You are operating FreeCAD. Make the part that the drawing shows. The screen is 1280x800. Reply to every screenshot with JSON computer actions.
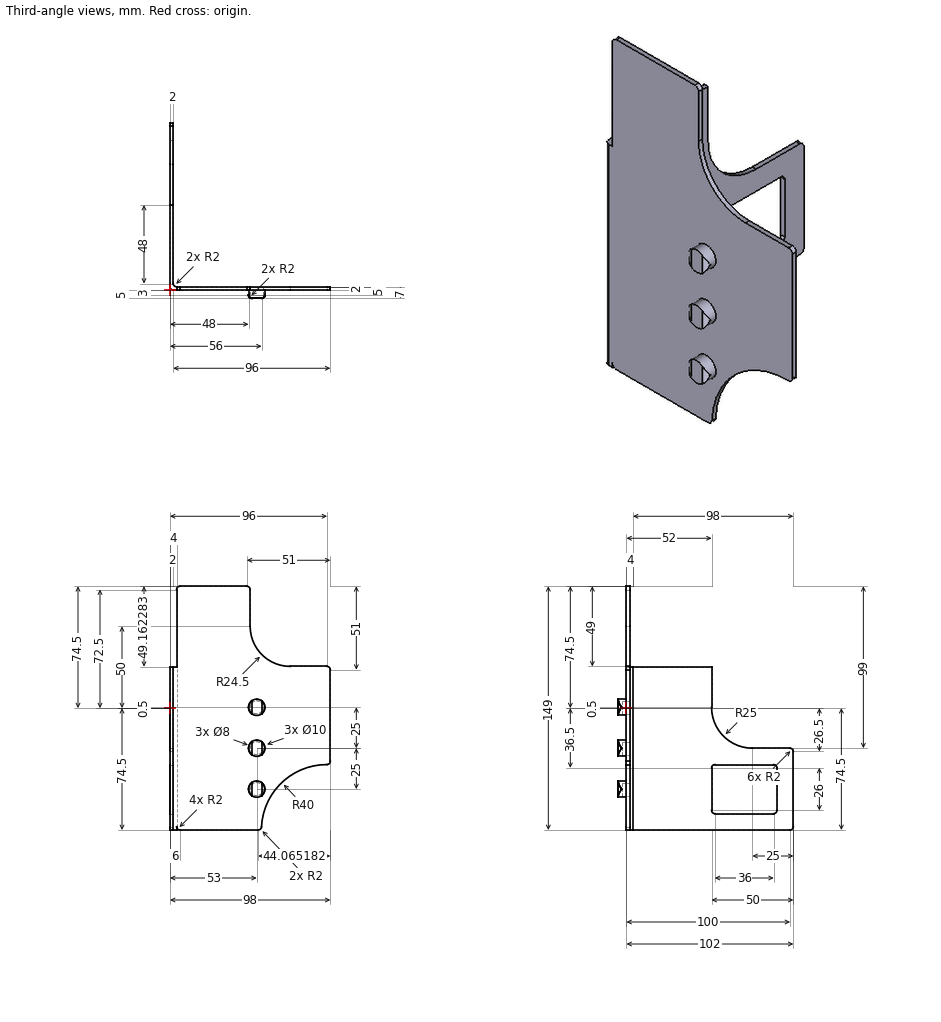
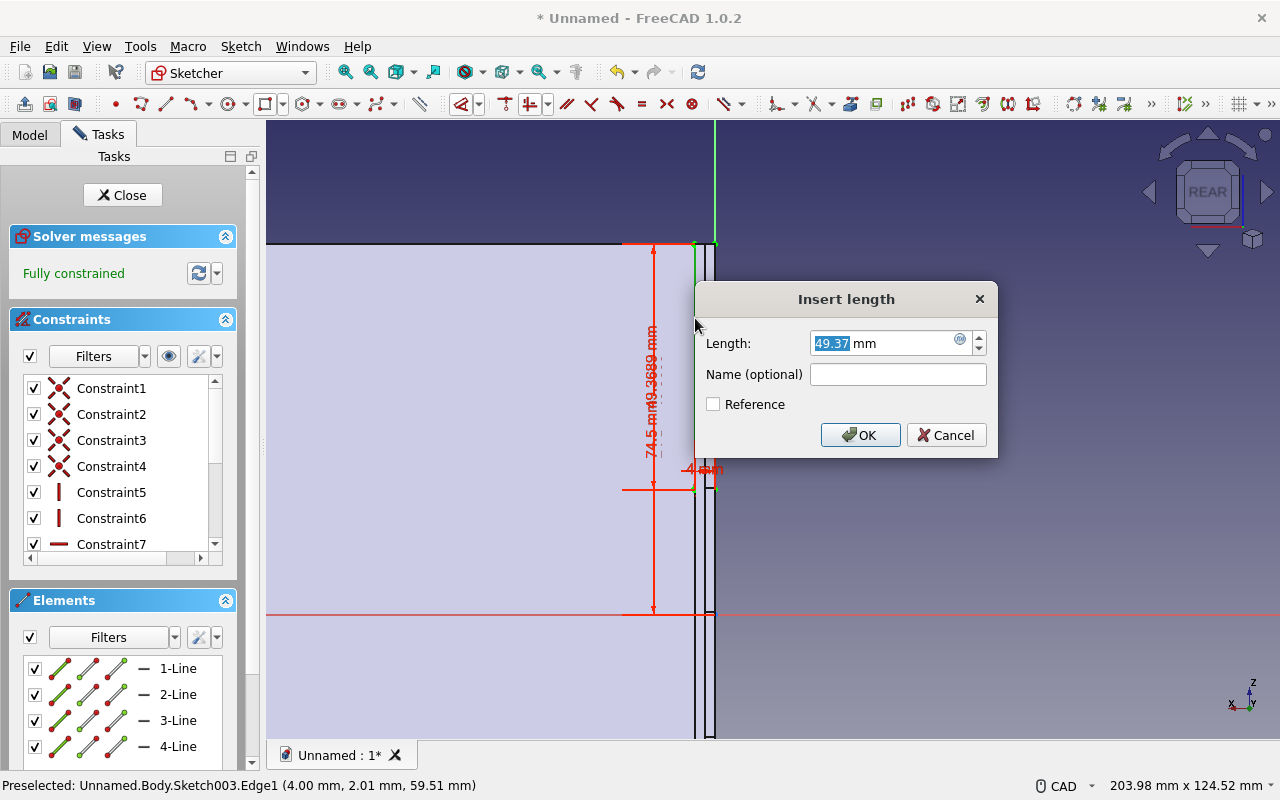
{"action": "type", "text": "49.162283"}
{"action": "key", "text": "Return"}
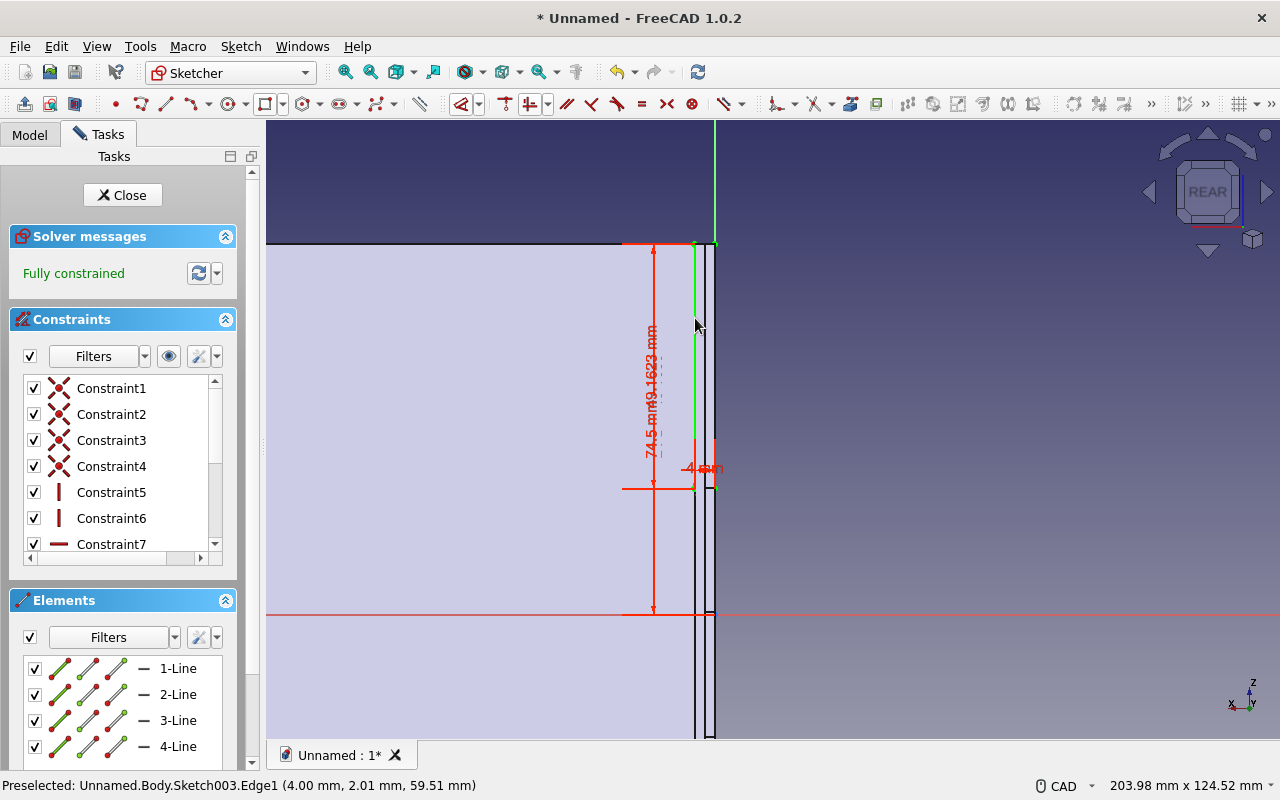
{"action": "left_click", "coordinate": [123, 195]}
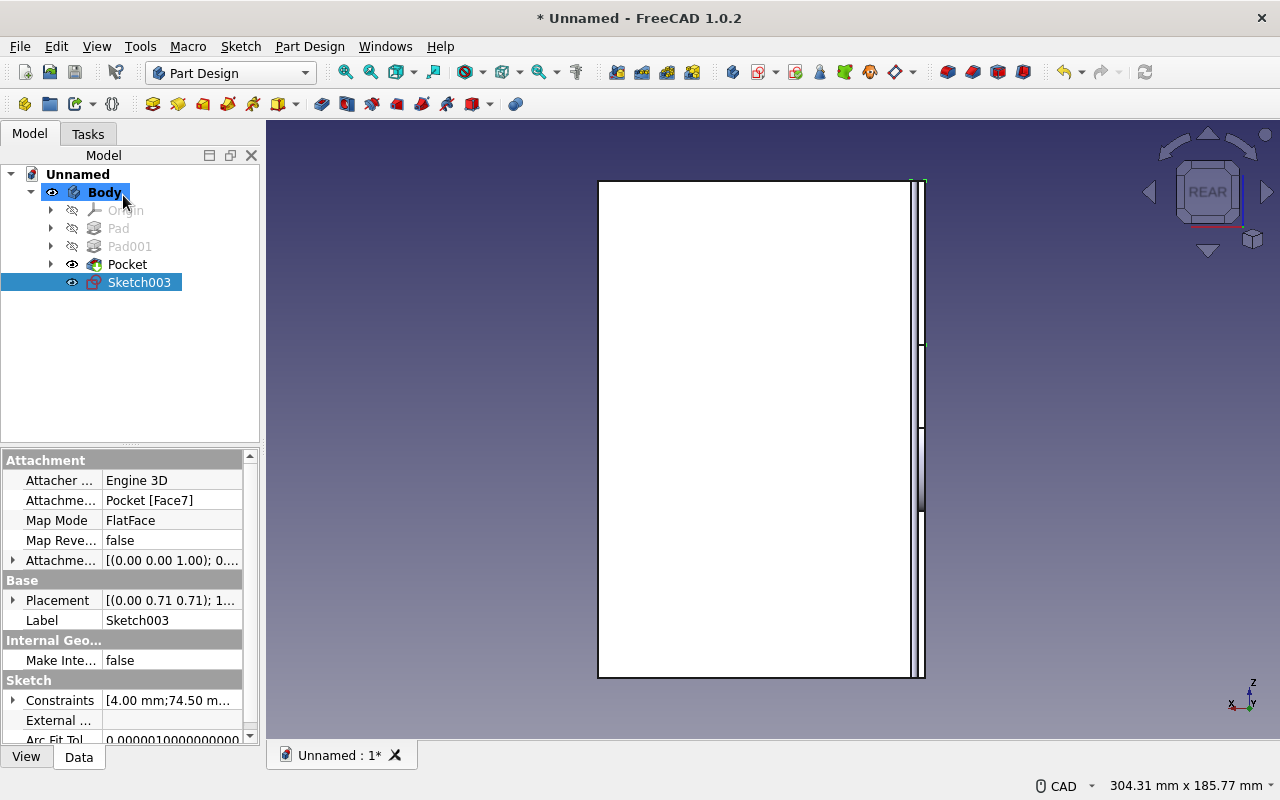
{"action": "left_click", "coordinate": [322, 104]}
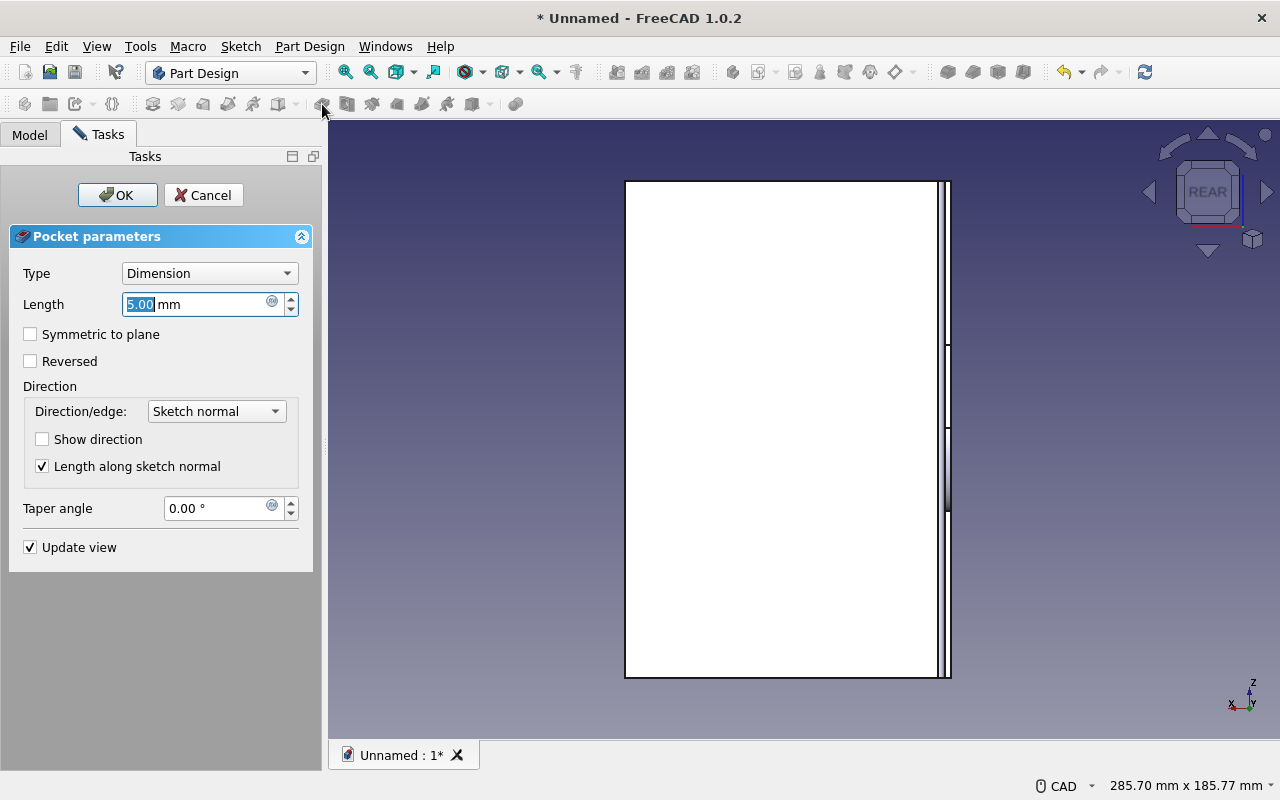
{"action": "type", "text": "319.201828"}
{"action": "key", "text": "Tab"}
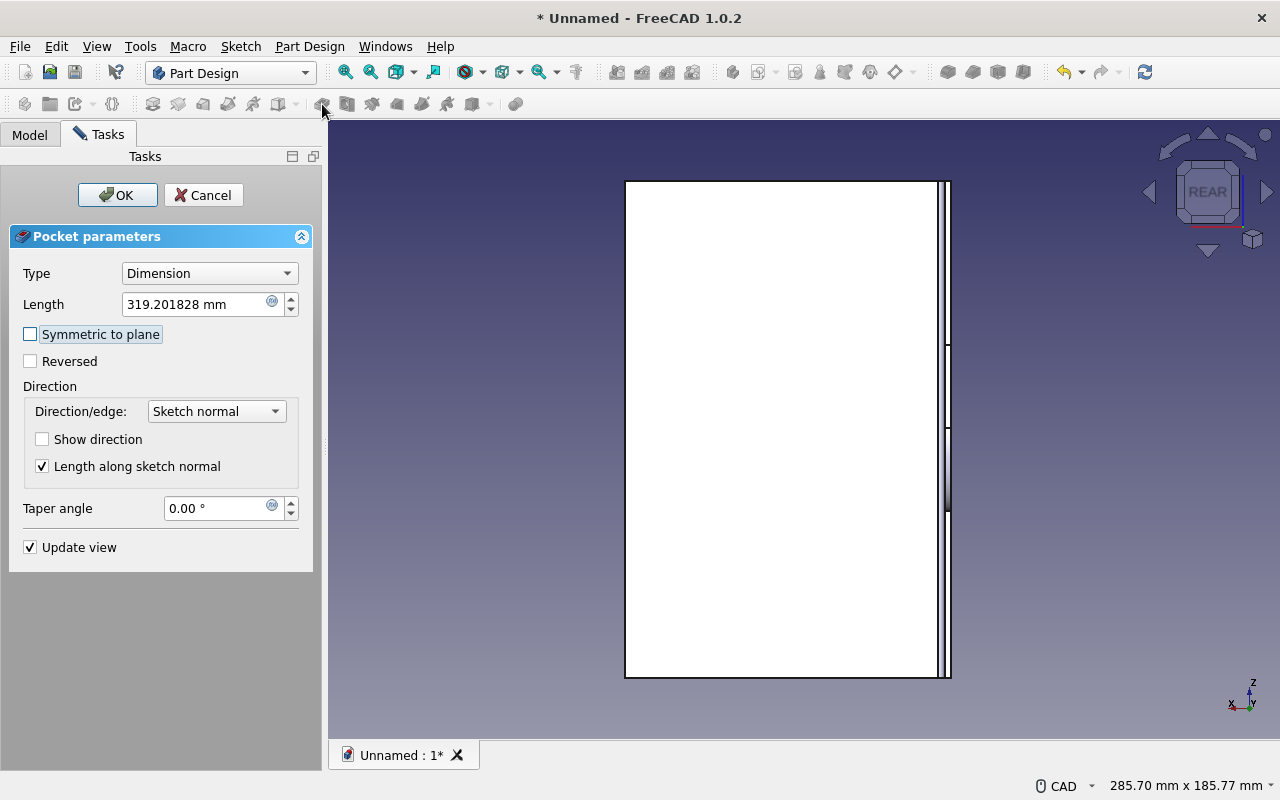
{"action": "left_click", "coordinate": [31, 334]}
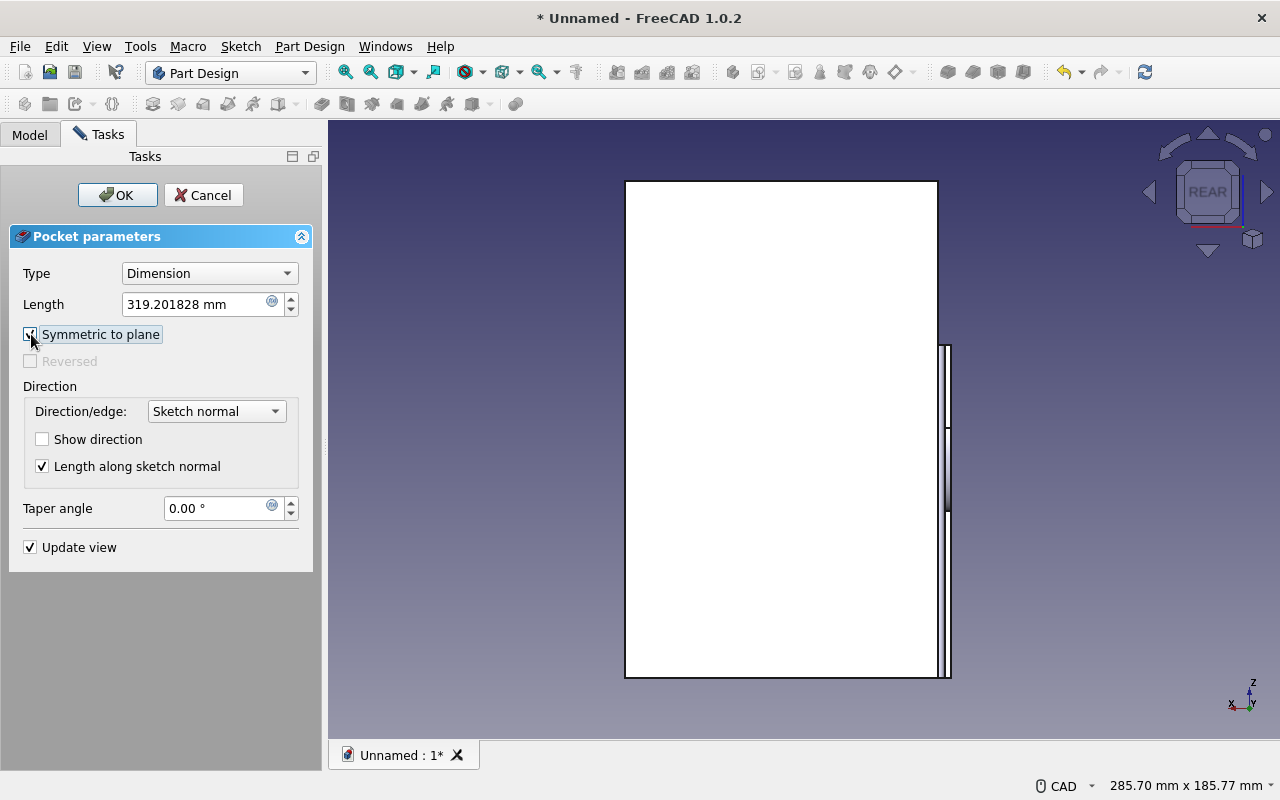
{"action": "left_click", "coordinate": [118, 195]}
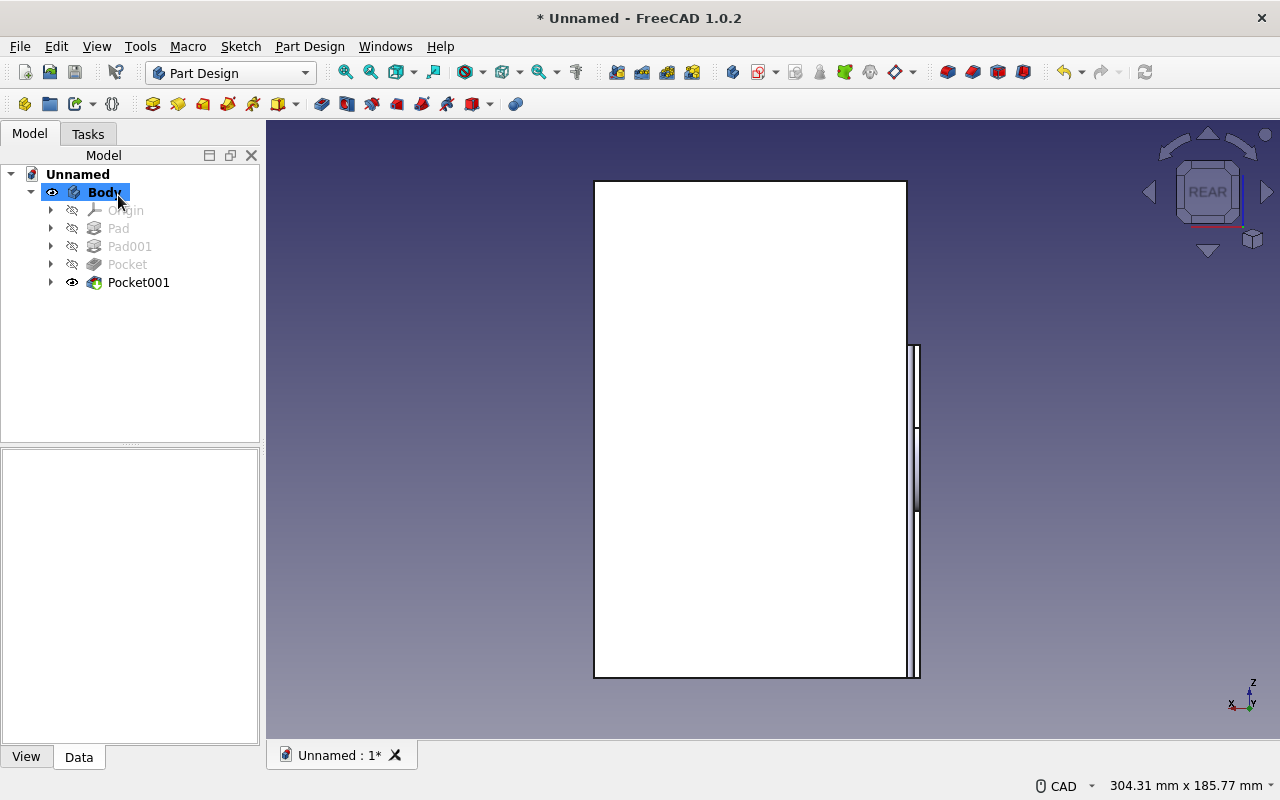
{"action": "key", "text": "0"}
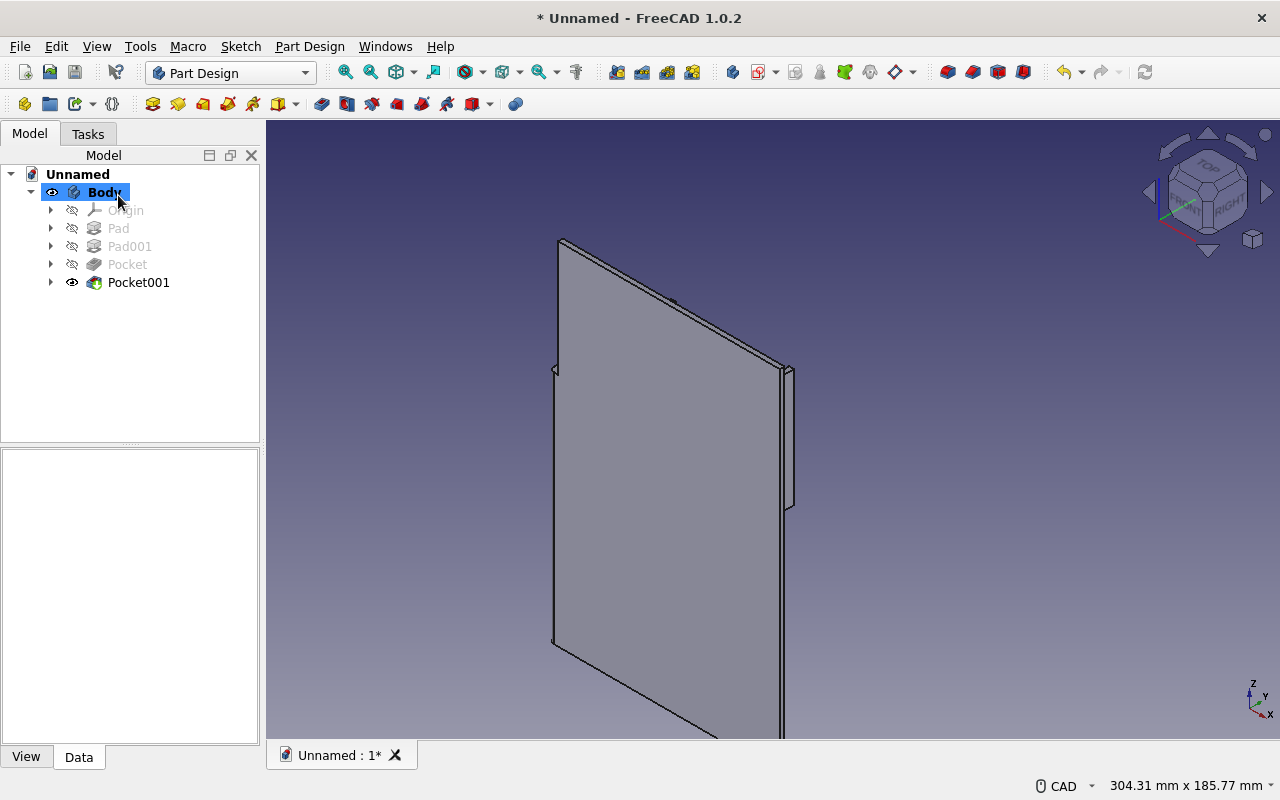
{"action": "key", "text": "v f"}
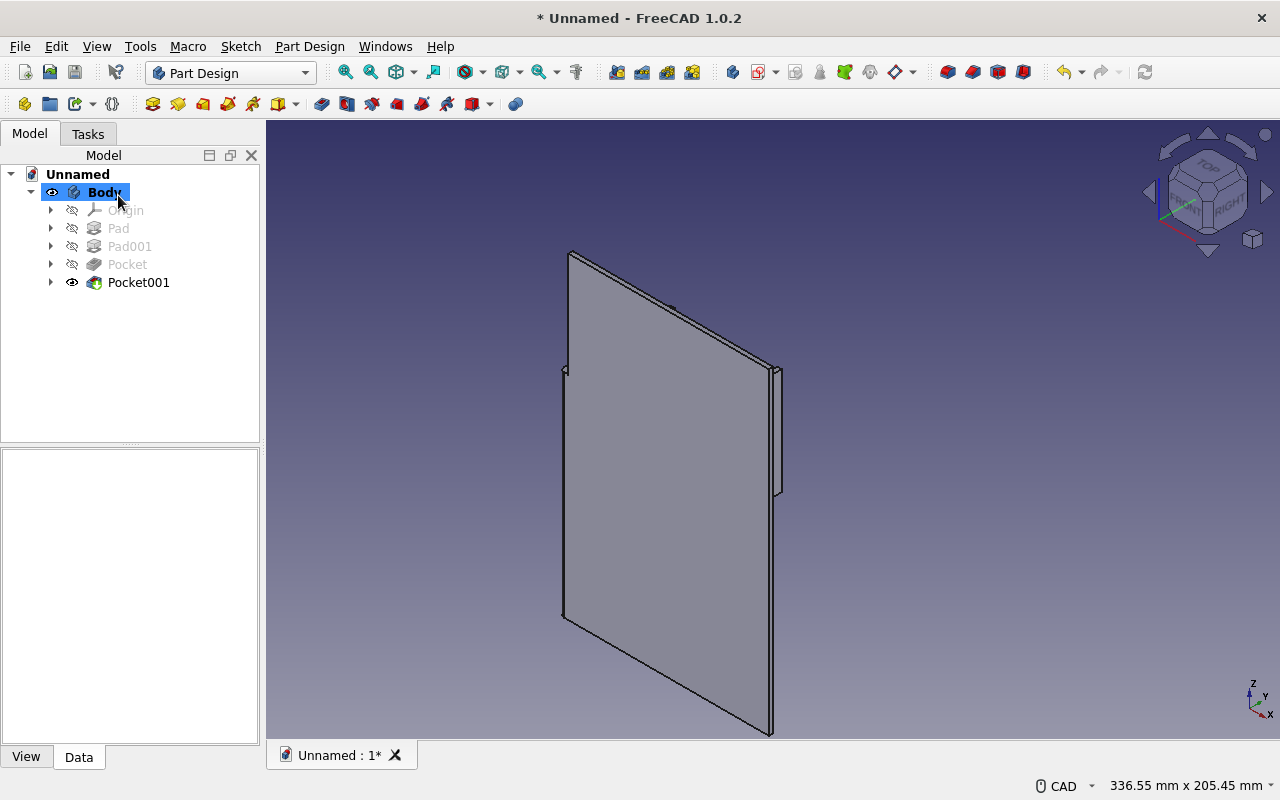
{"action": "key", "text": "3"}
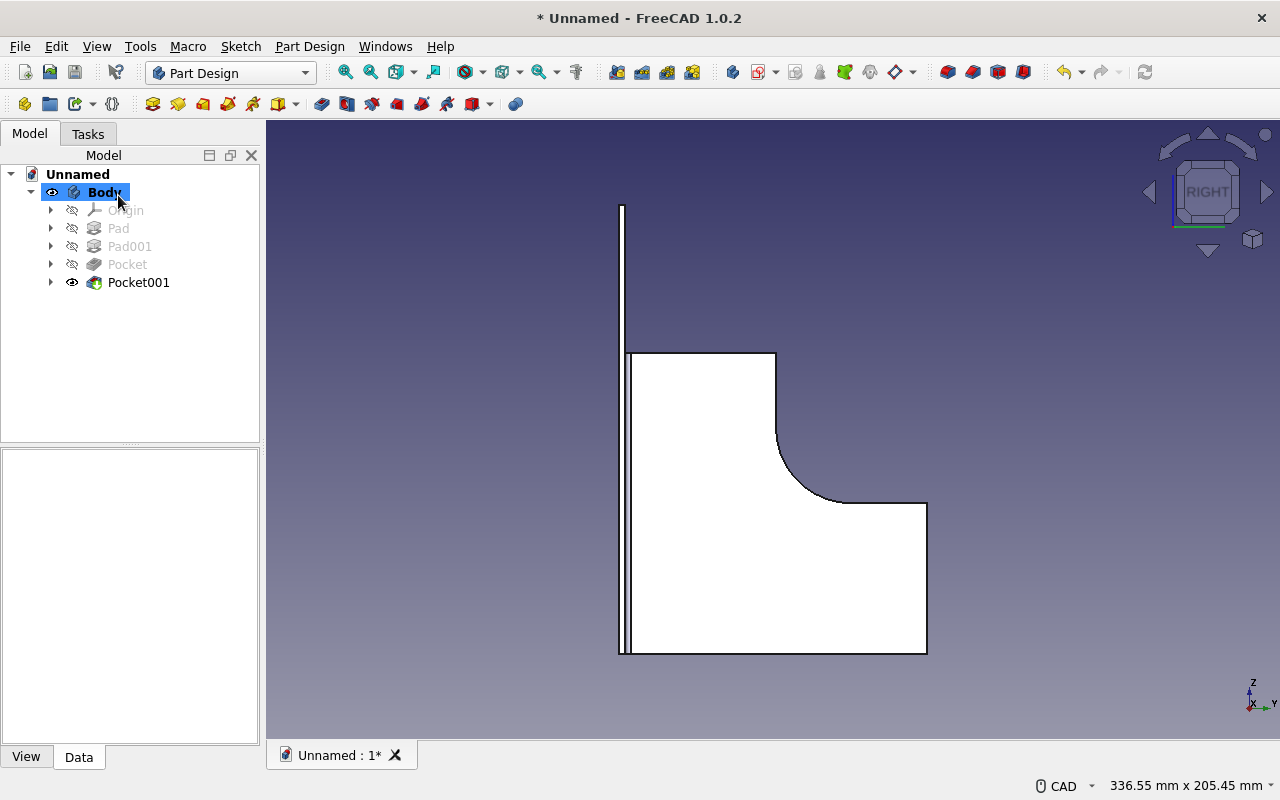
{"action": "left_click", "coordinate": [737, 546]}